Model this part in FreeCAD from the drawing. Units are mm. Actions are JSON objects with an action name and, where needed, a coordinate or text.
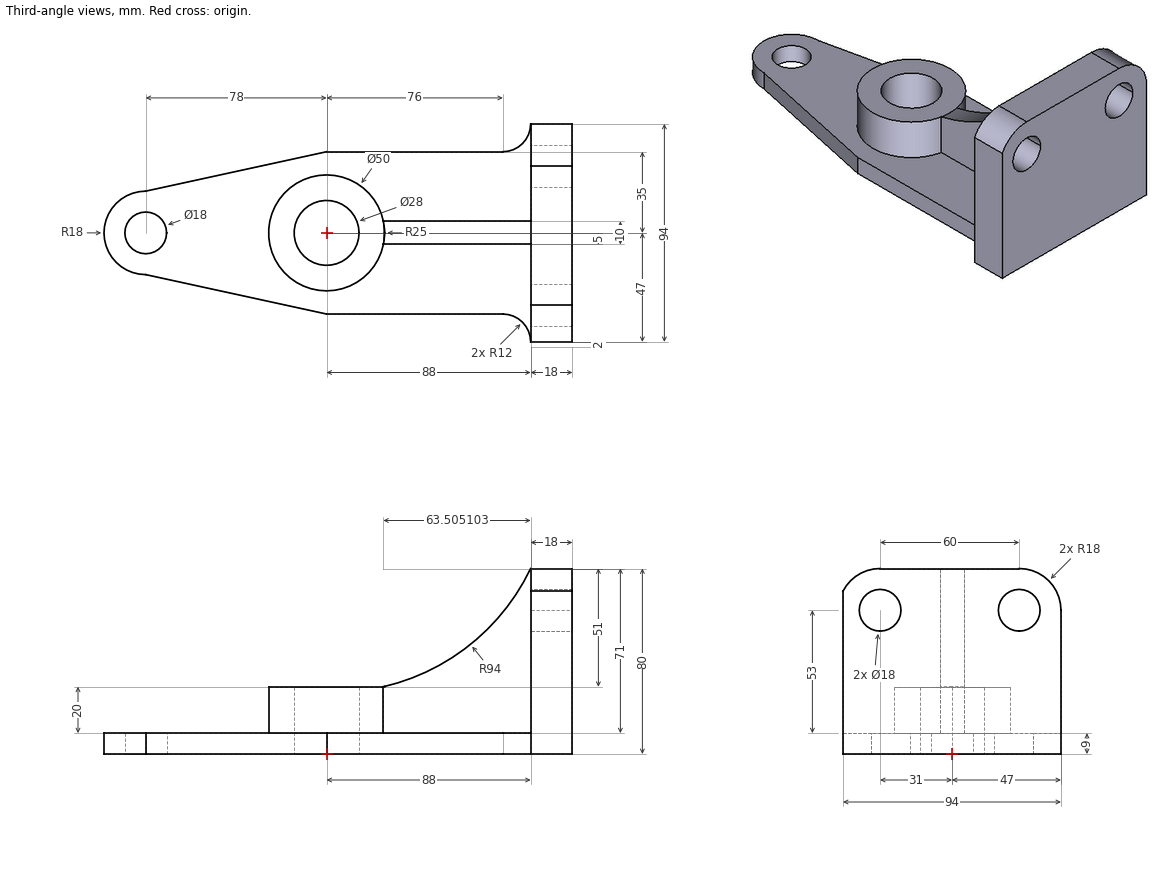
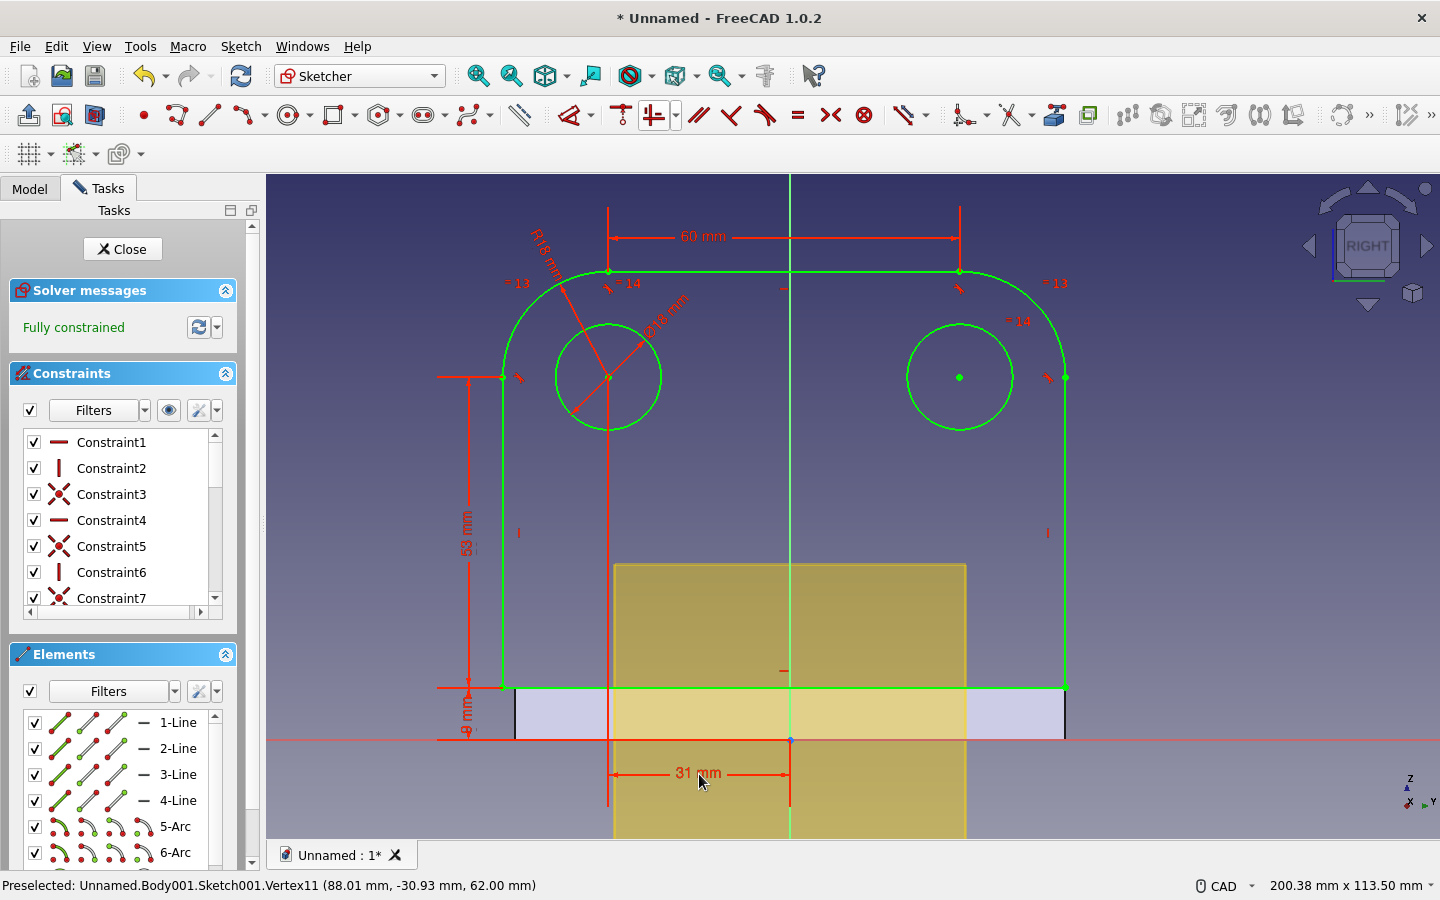
{"action": "left_click", "coordinate": [123, 249]}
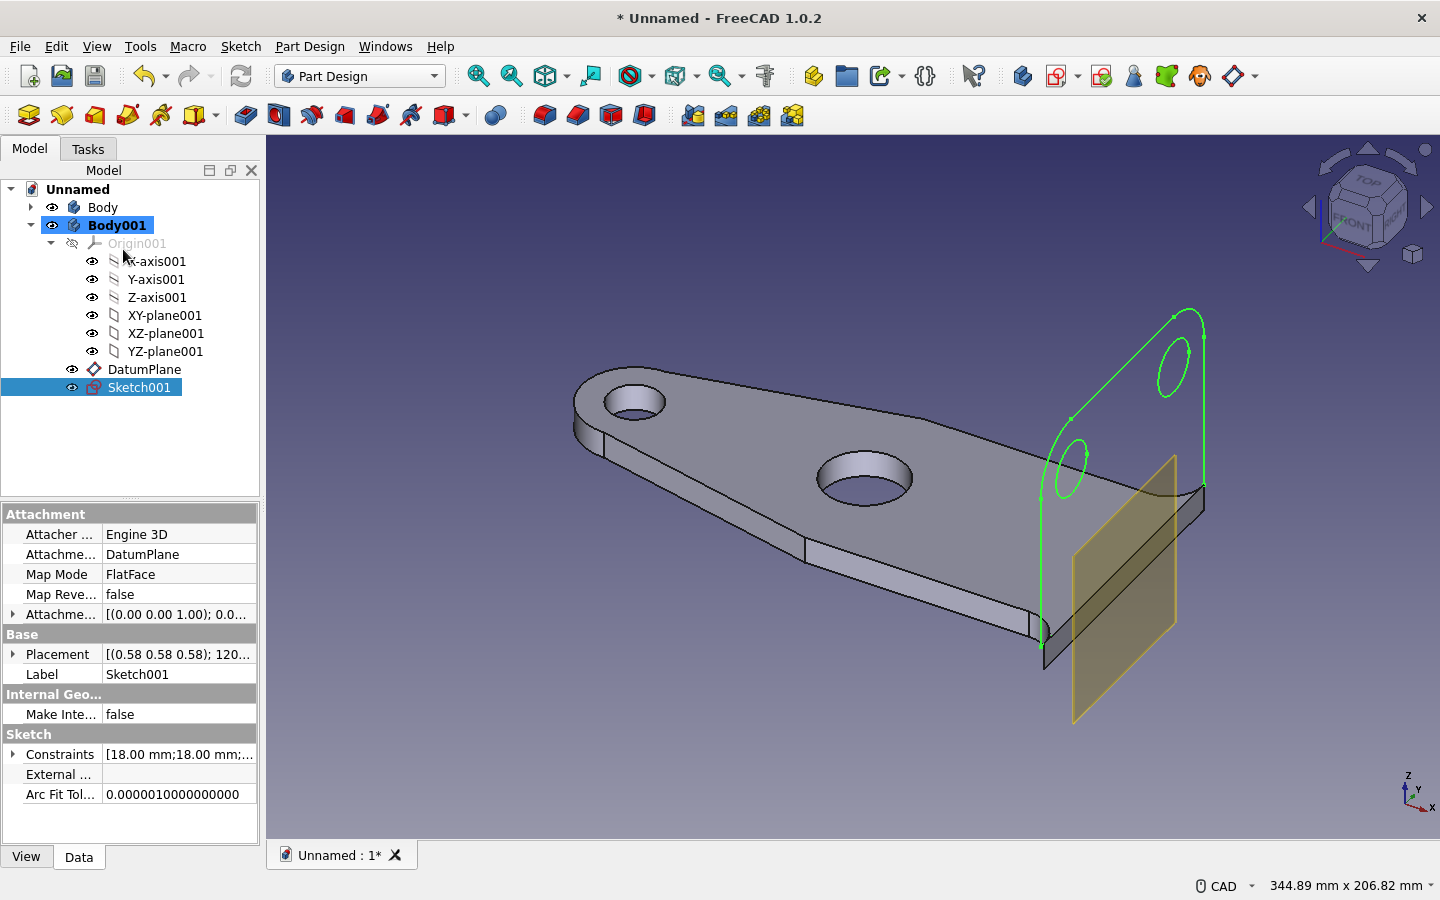
{"action": "left_click", "coordinate": [29, 116]}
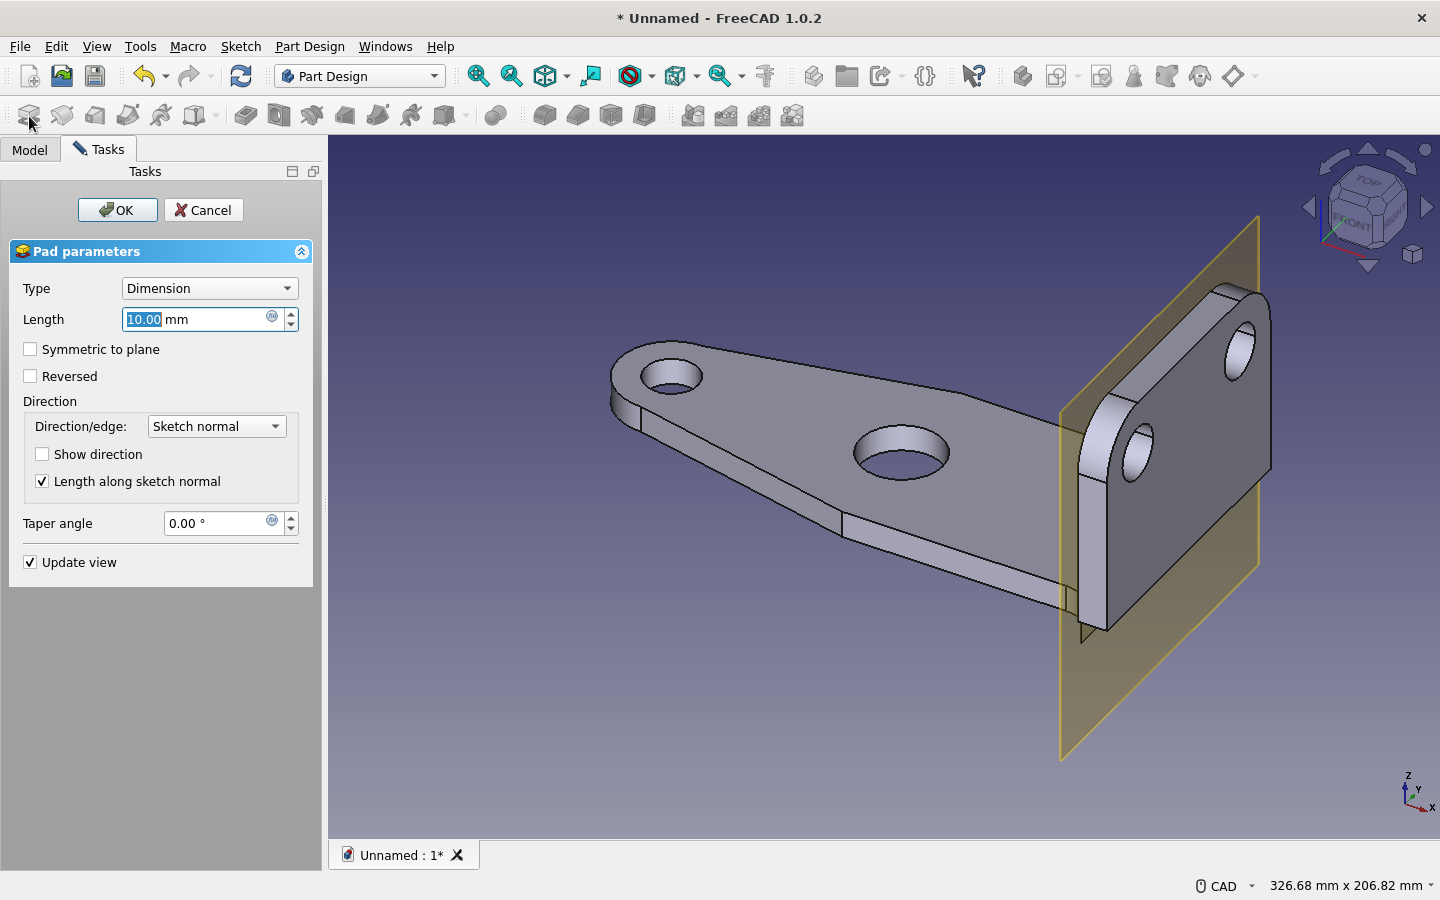
{"action": "type", "text": "18"}
{"action": "key", "text": "Tab"}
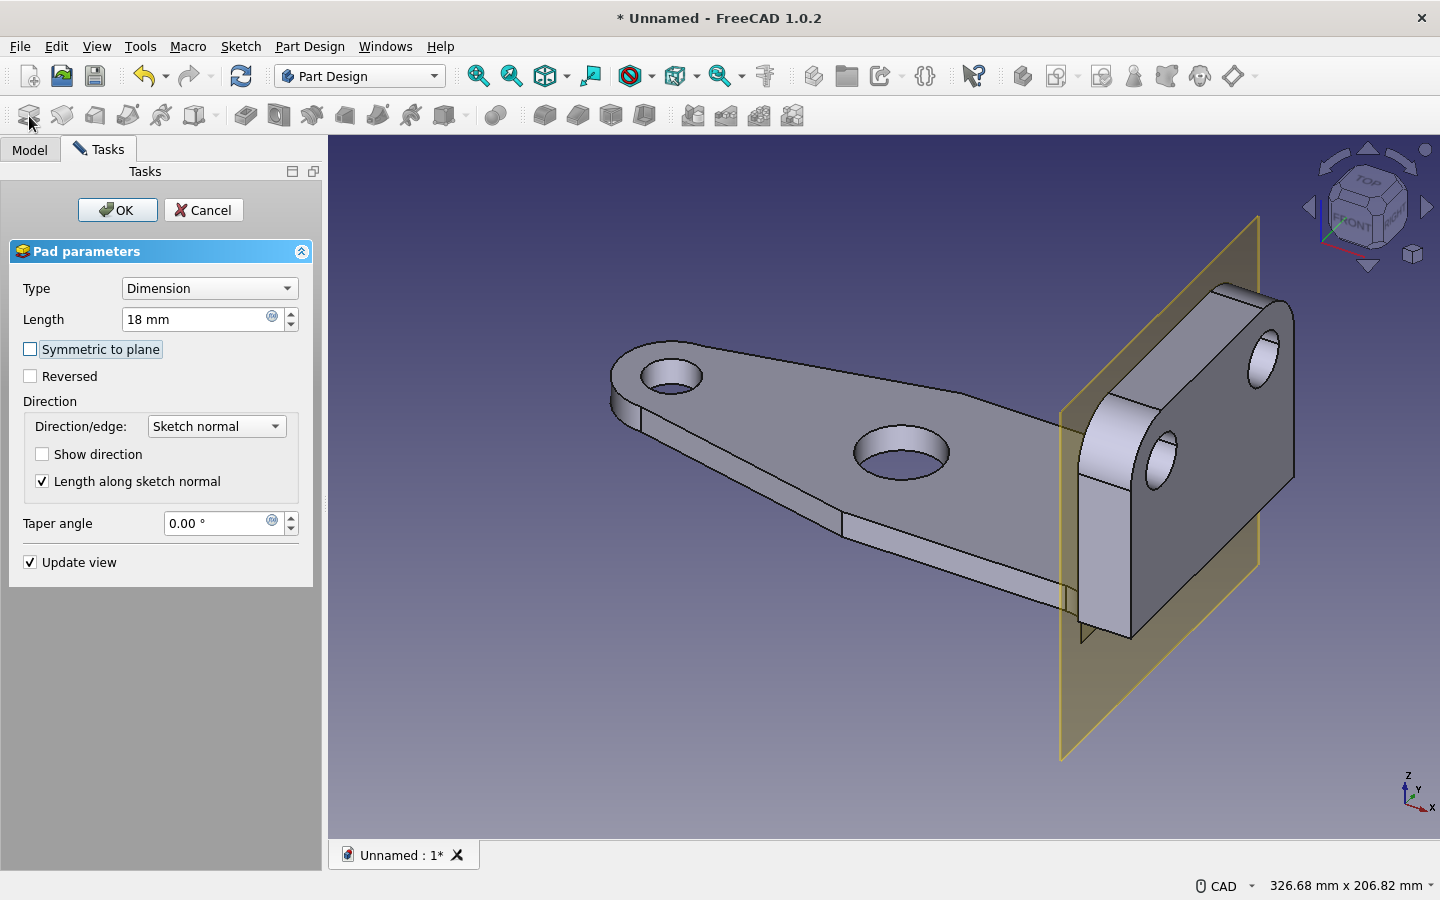
{"action": "left_click", "coordinate": [118, 210]}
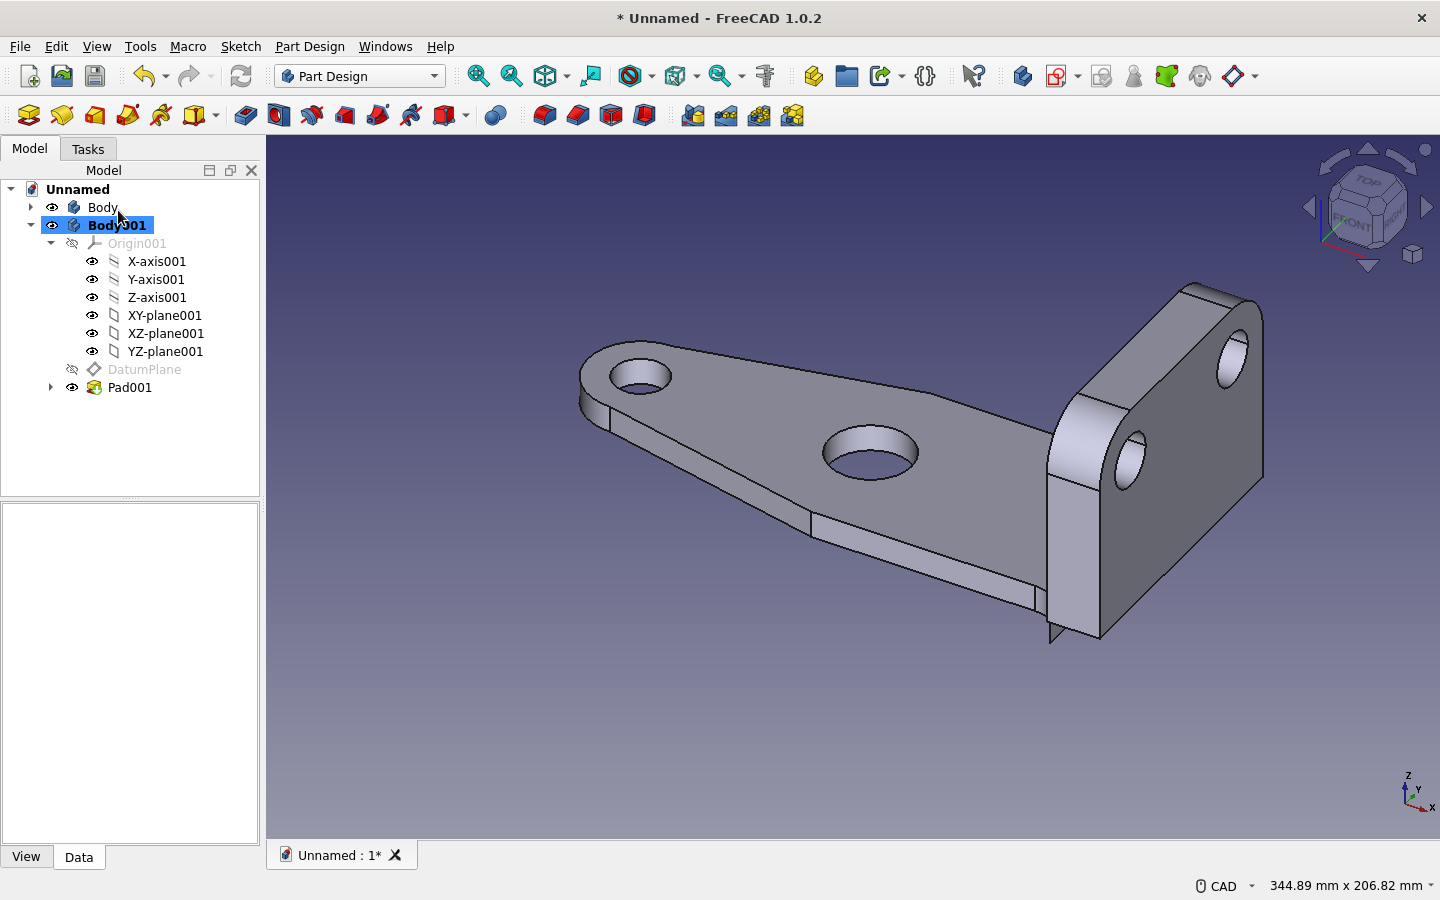
{"action": "double_click", "coordinate": [97, 207]}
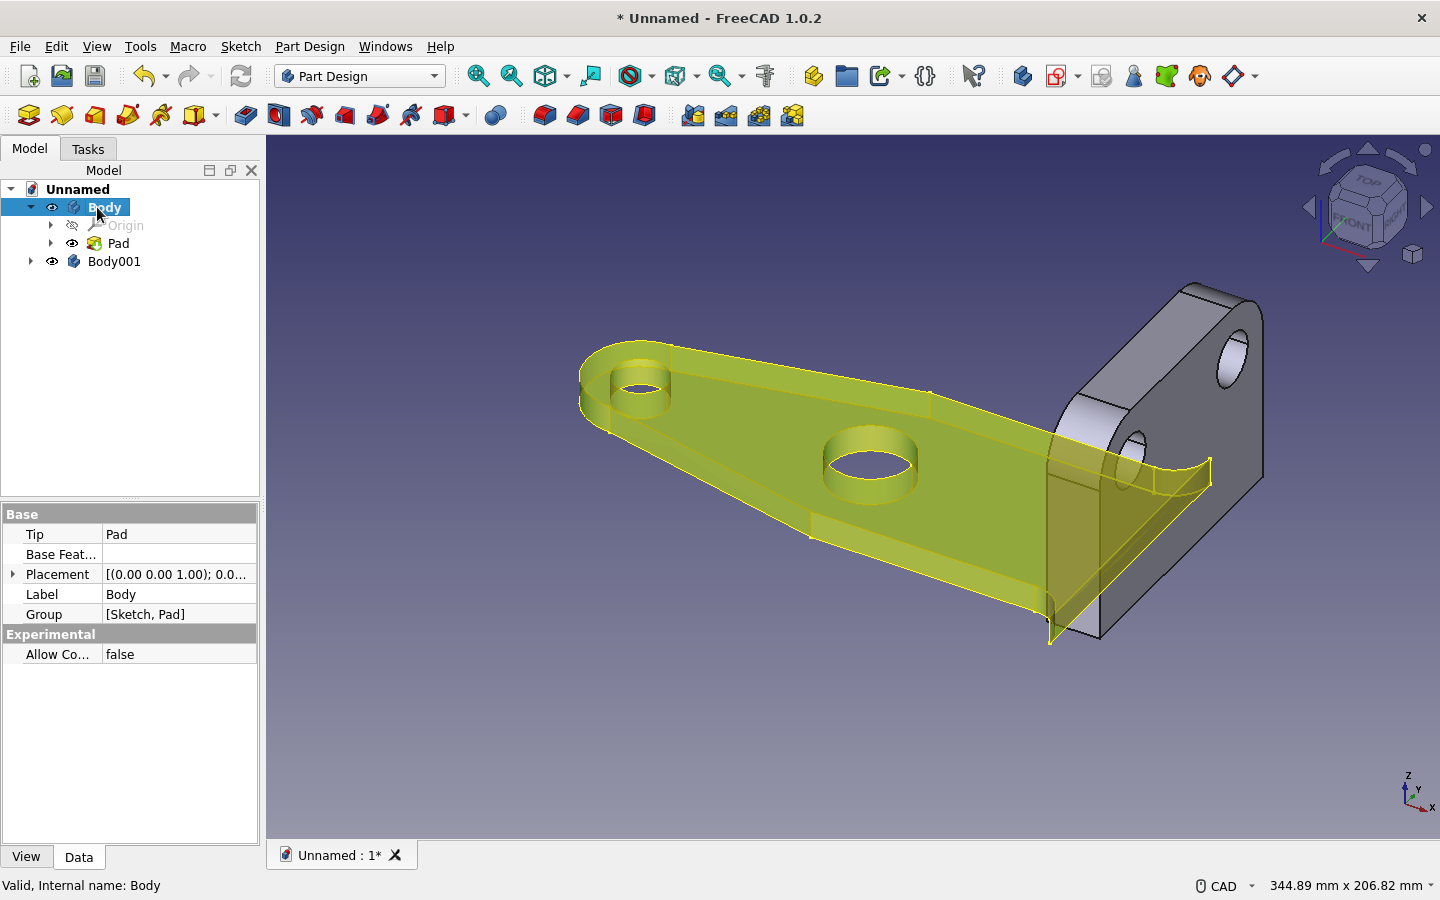
{"action": "left_click", "coordinate": [97, 207]}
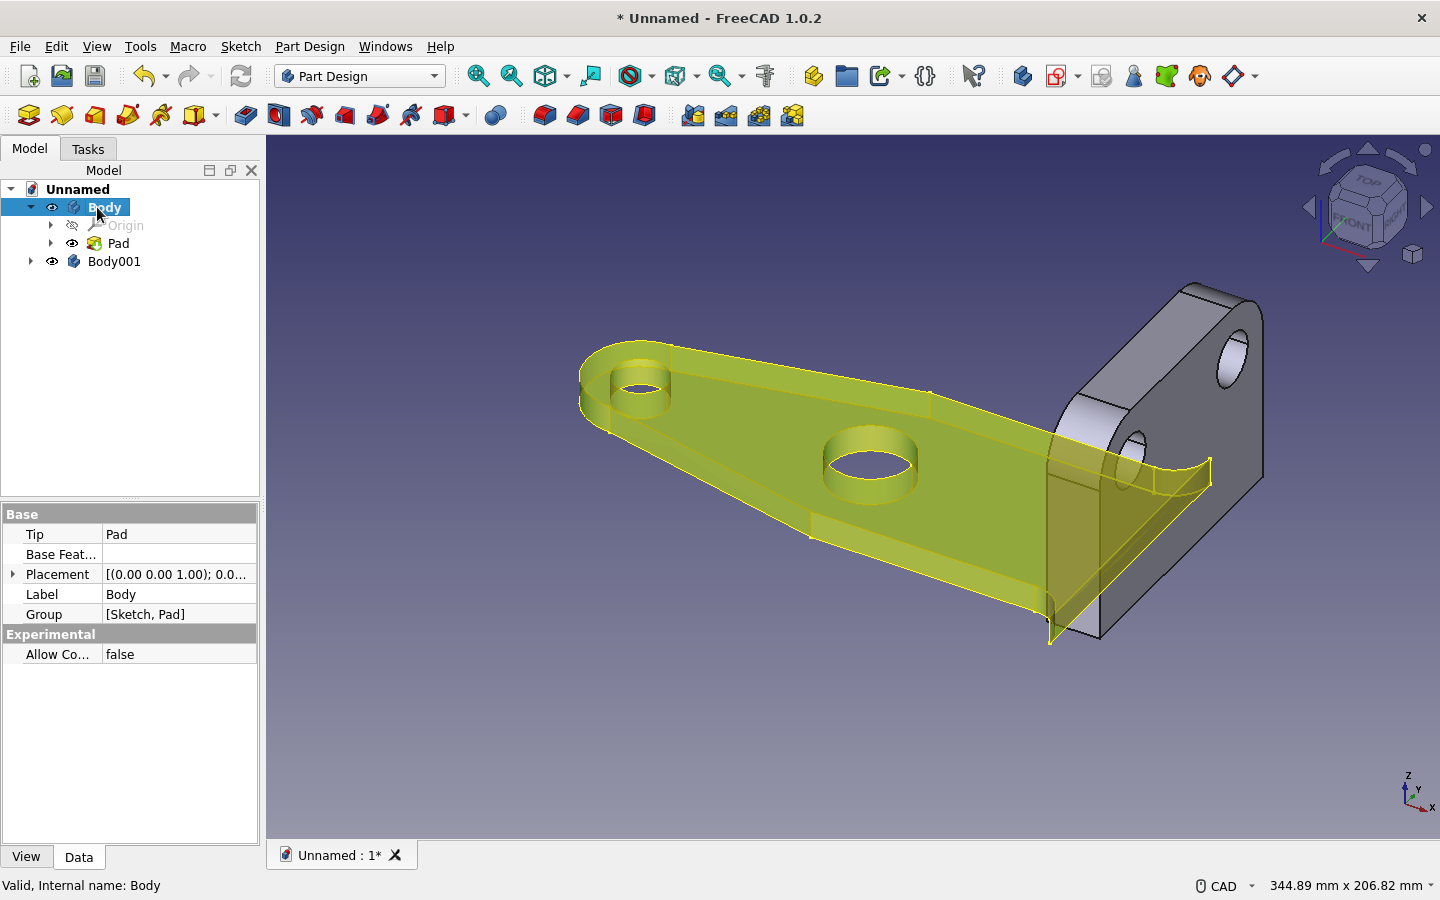
{"action": "left_click", "coordinate": [148, 654]}